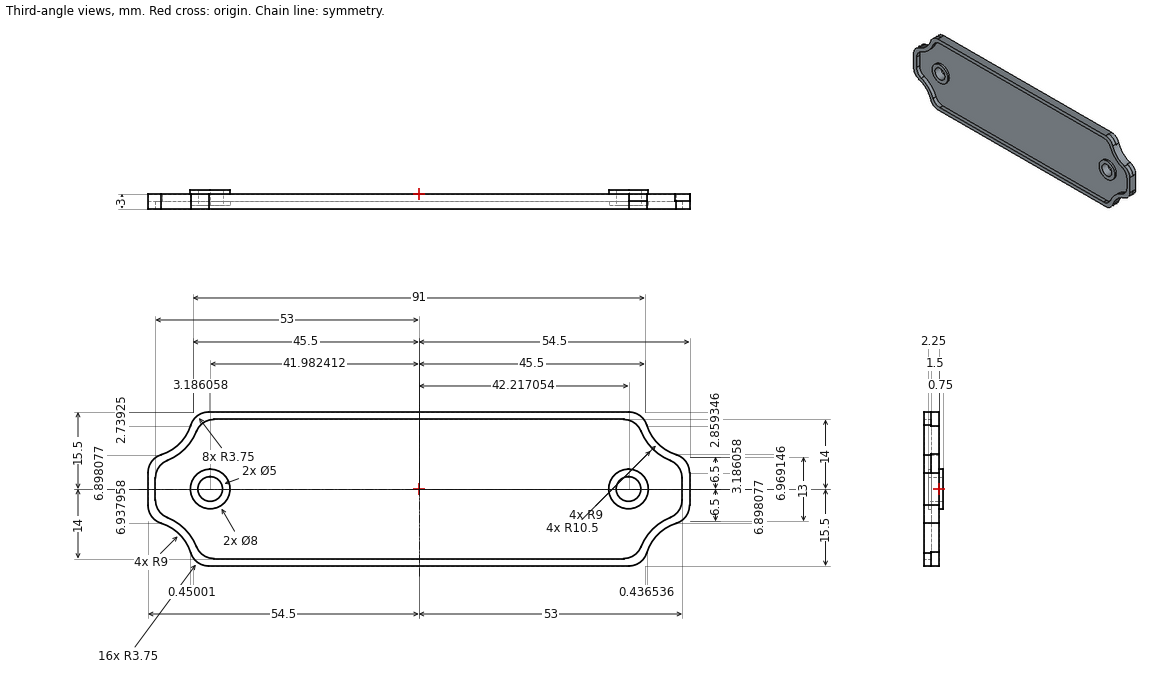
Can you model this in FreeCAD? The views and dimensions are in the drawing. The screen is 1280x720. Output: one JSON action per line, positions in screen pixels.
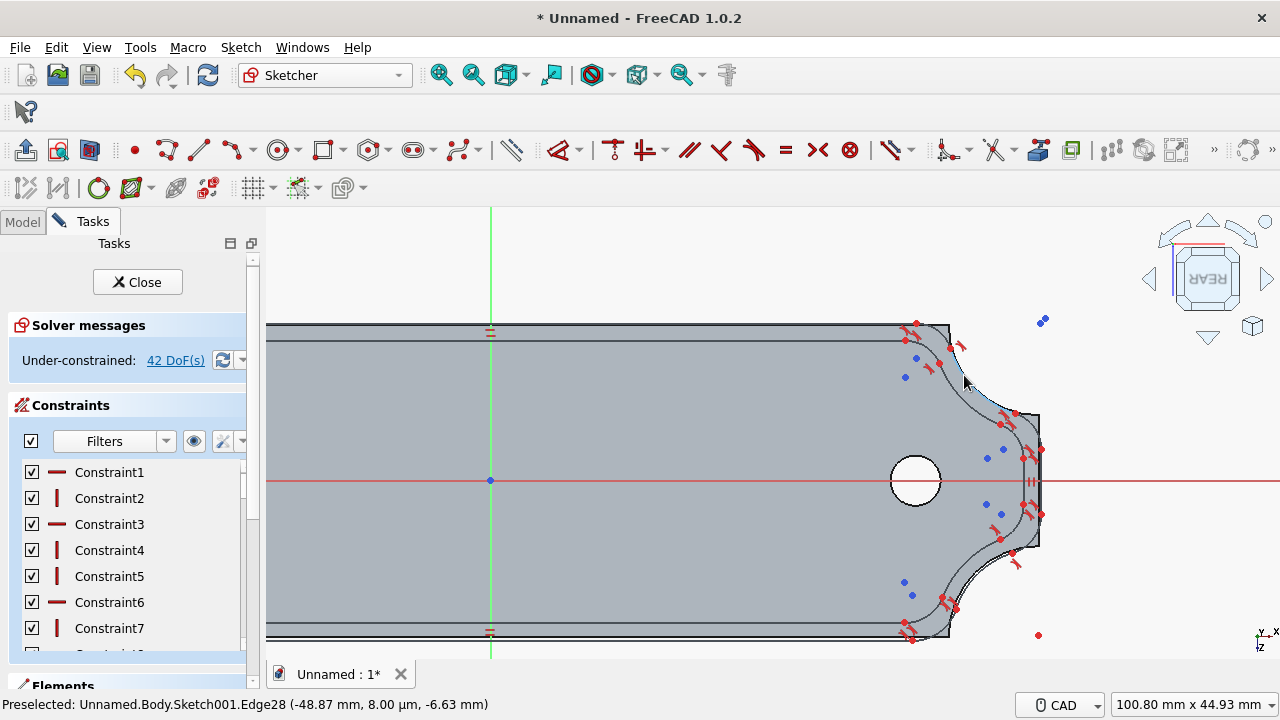
{"action": "left_click", "coordinate": [963, 374]}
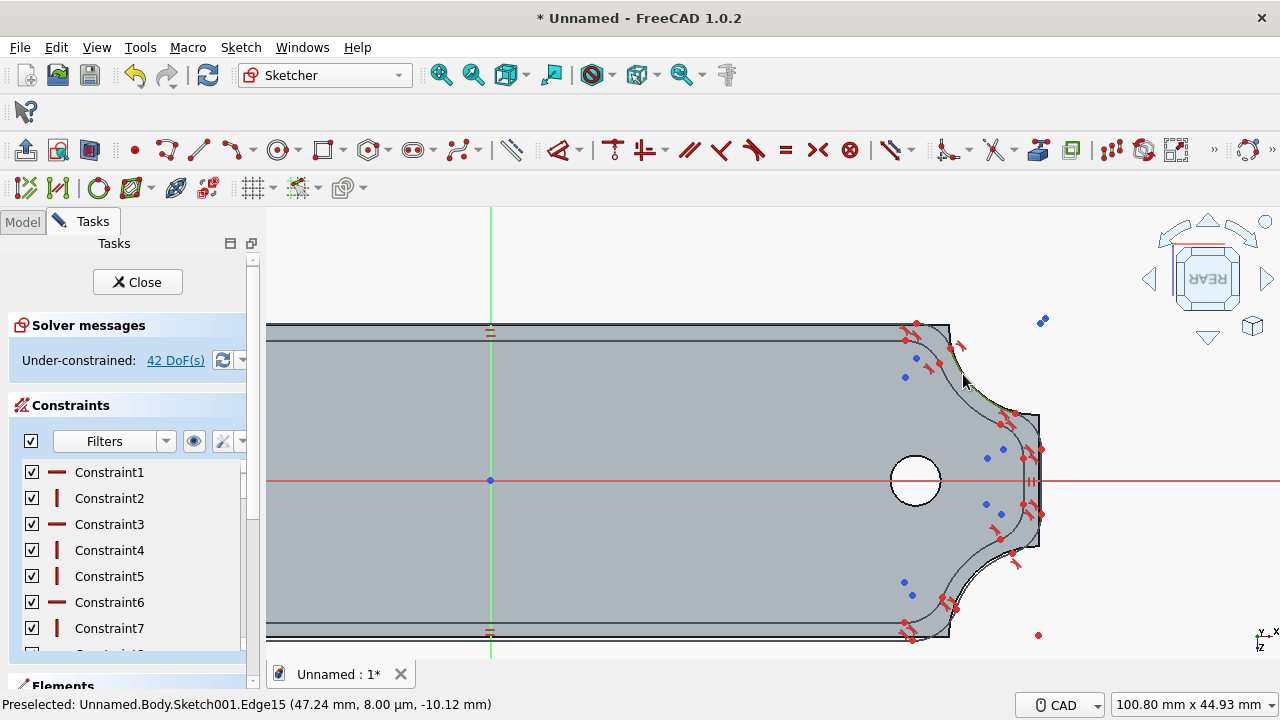
{"action": "left_click", "coordinate": [952, 387]}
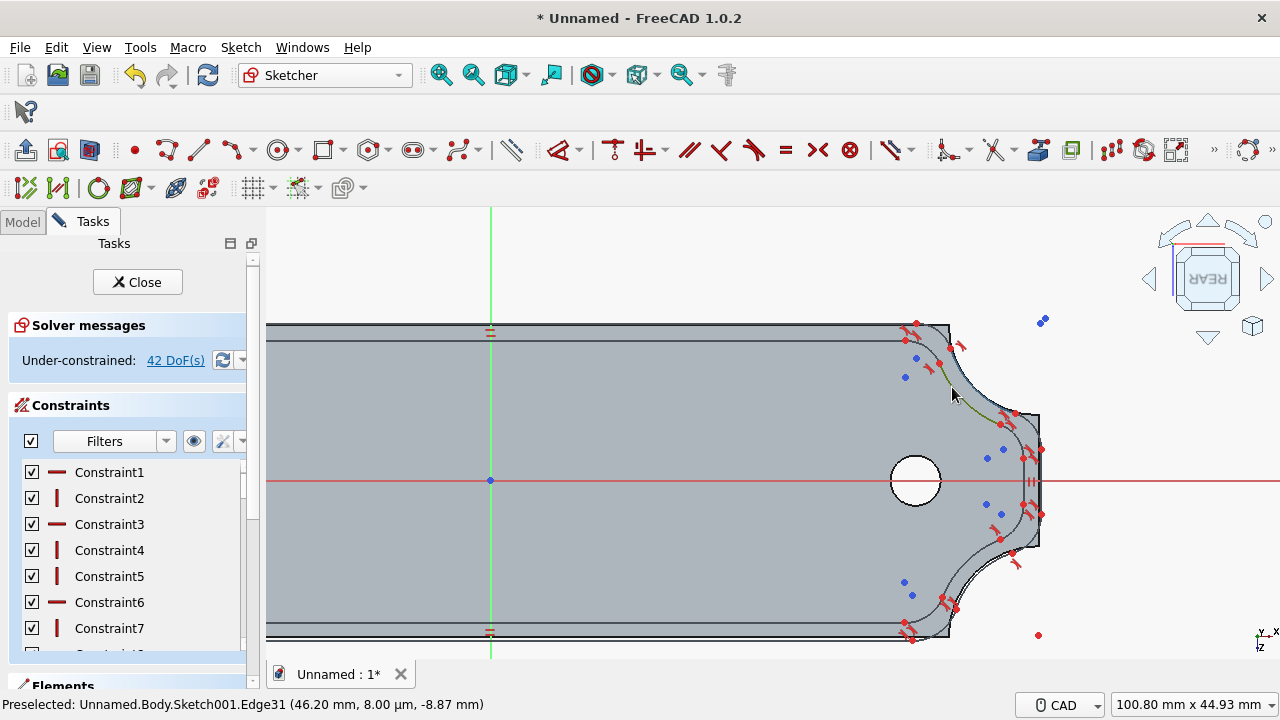
{"action": "left_click", "coordinate": [614, 150]}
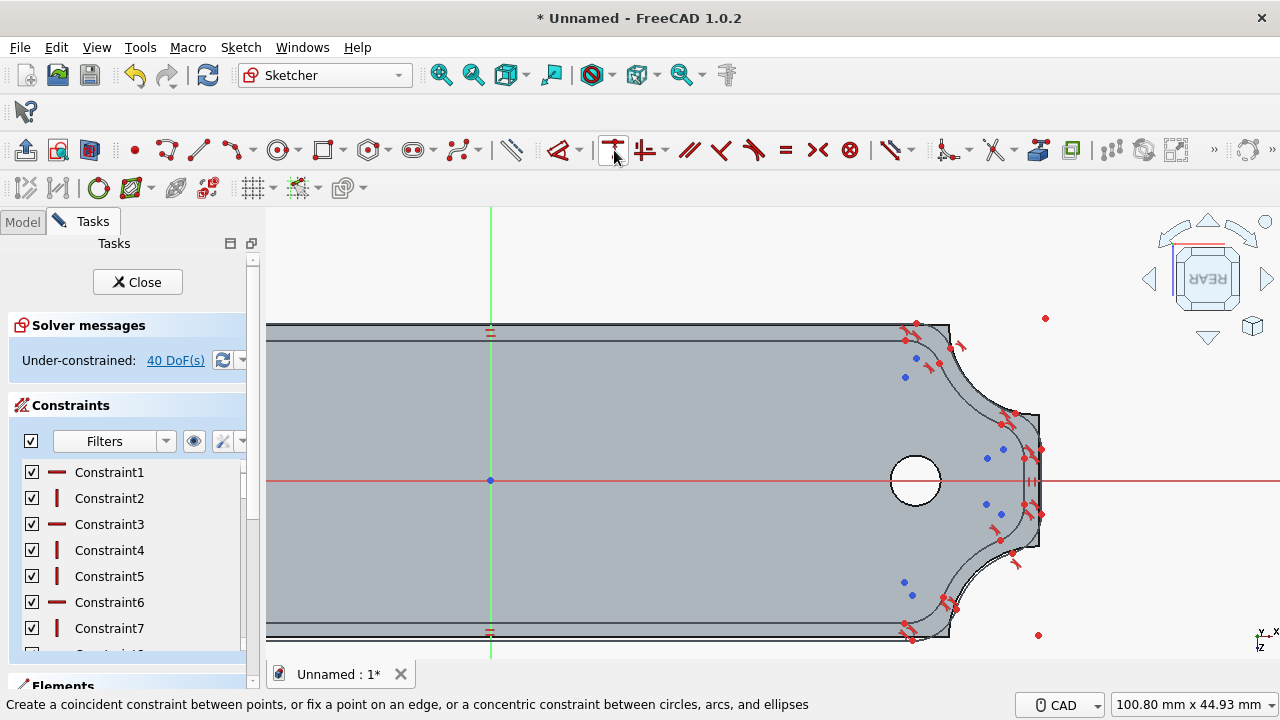
{"action": "scroll", "coordinate": [964, 375], "scroll_direction": "down", "scroll_amount": 3}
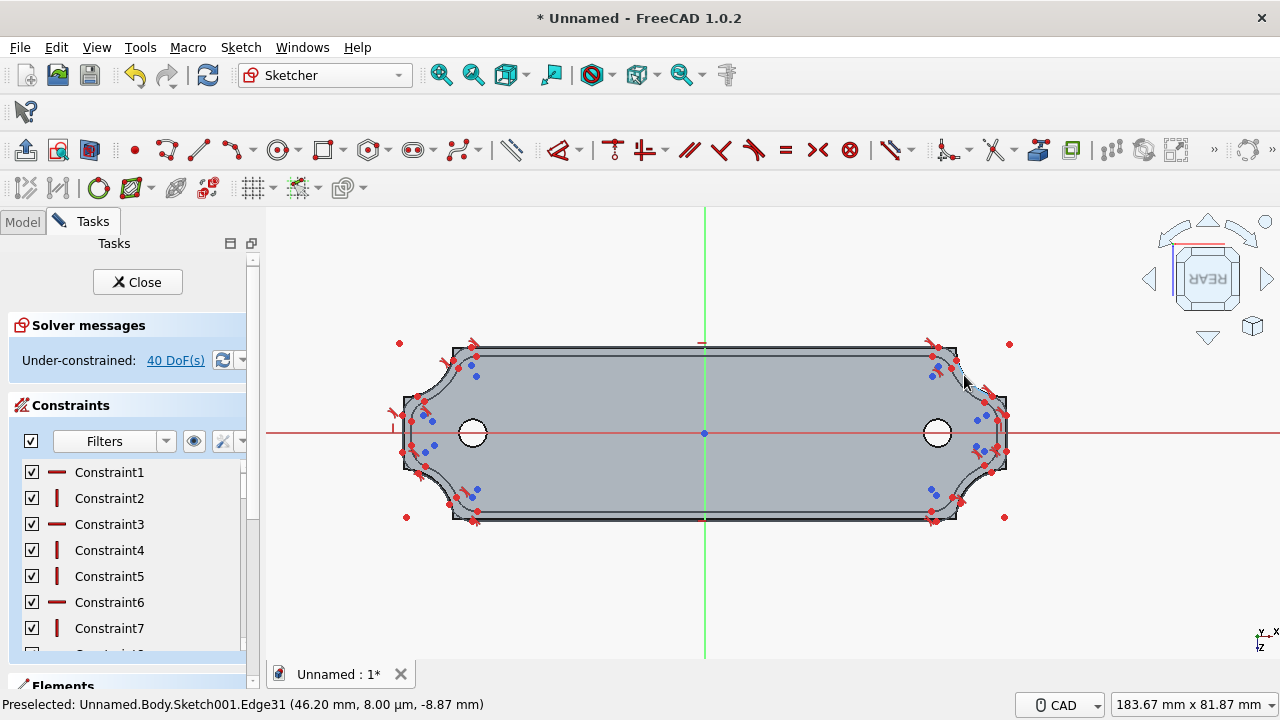
{"action": "scroll", "coordinate": [464, 348], "scroll_direction": "up", "scroll_amount": 4}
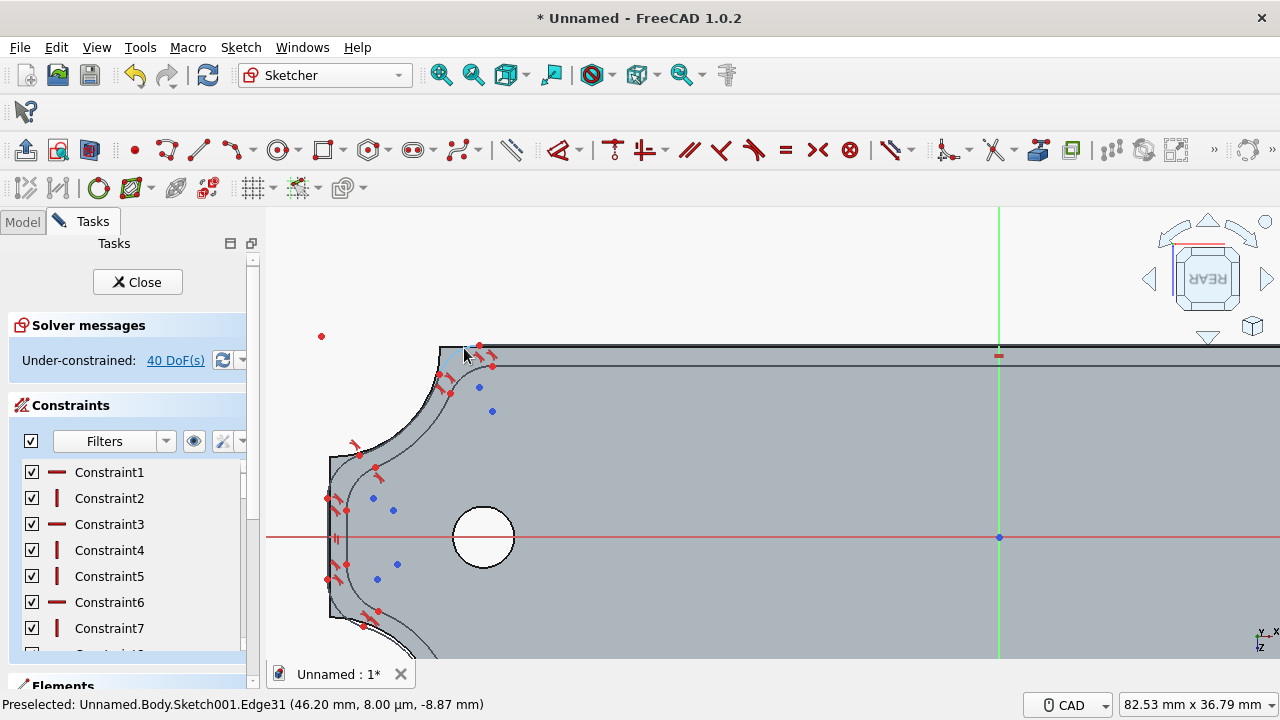
{"action": "left_click", "coordinate": [464, 348]}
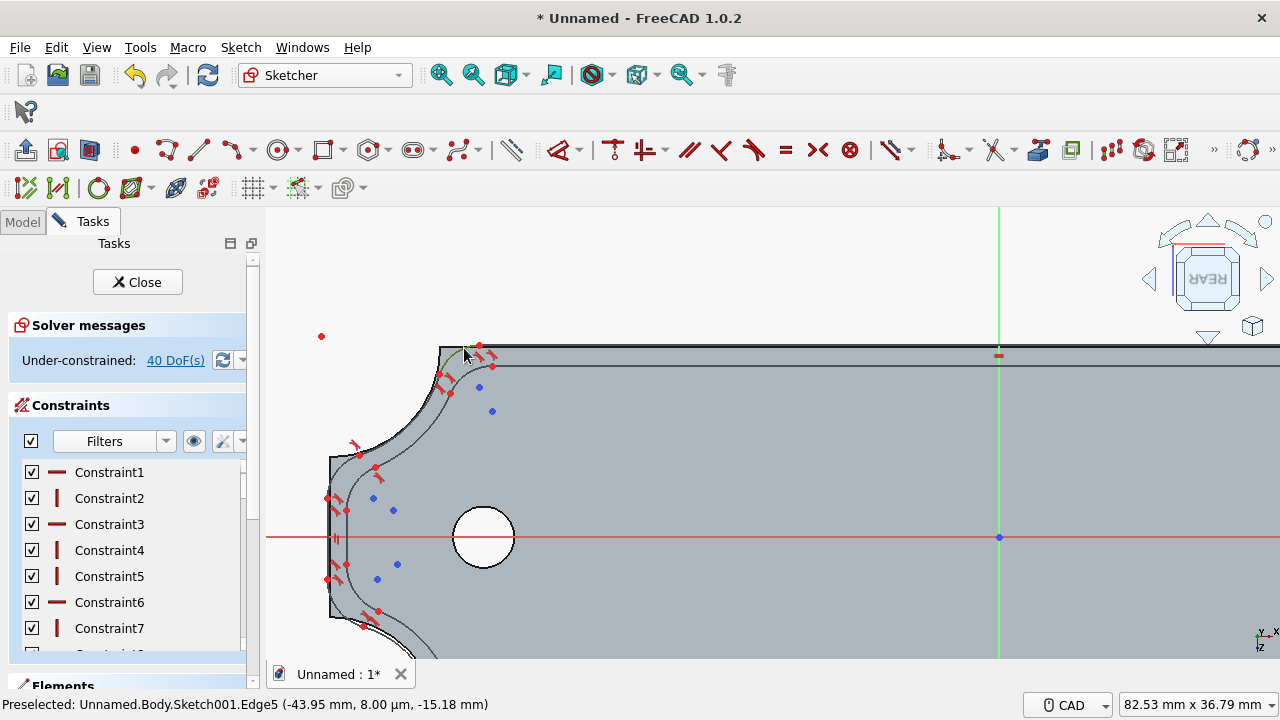
{"action": "left_click", "coordinate": [344, 463]}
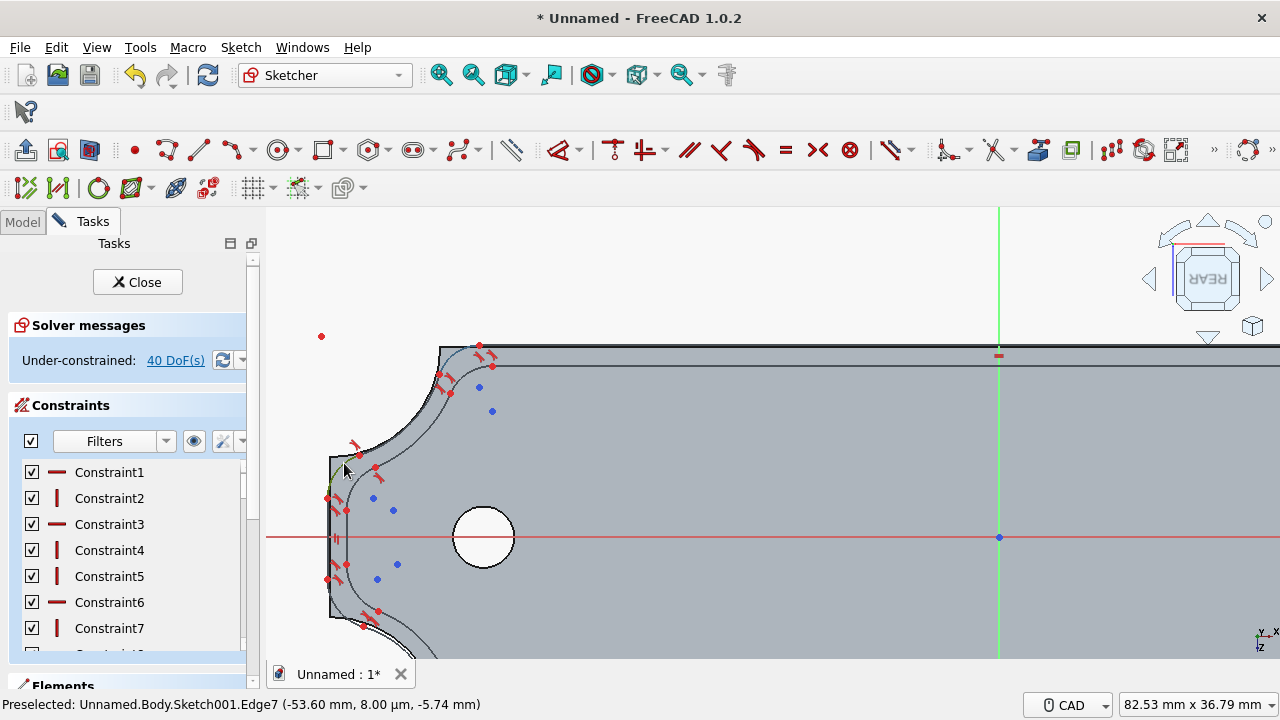
{"action": "left_click", "coordinate": [331, 598]}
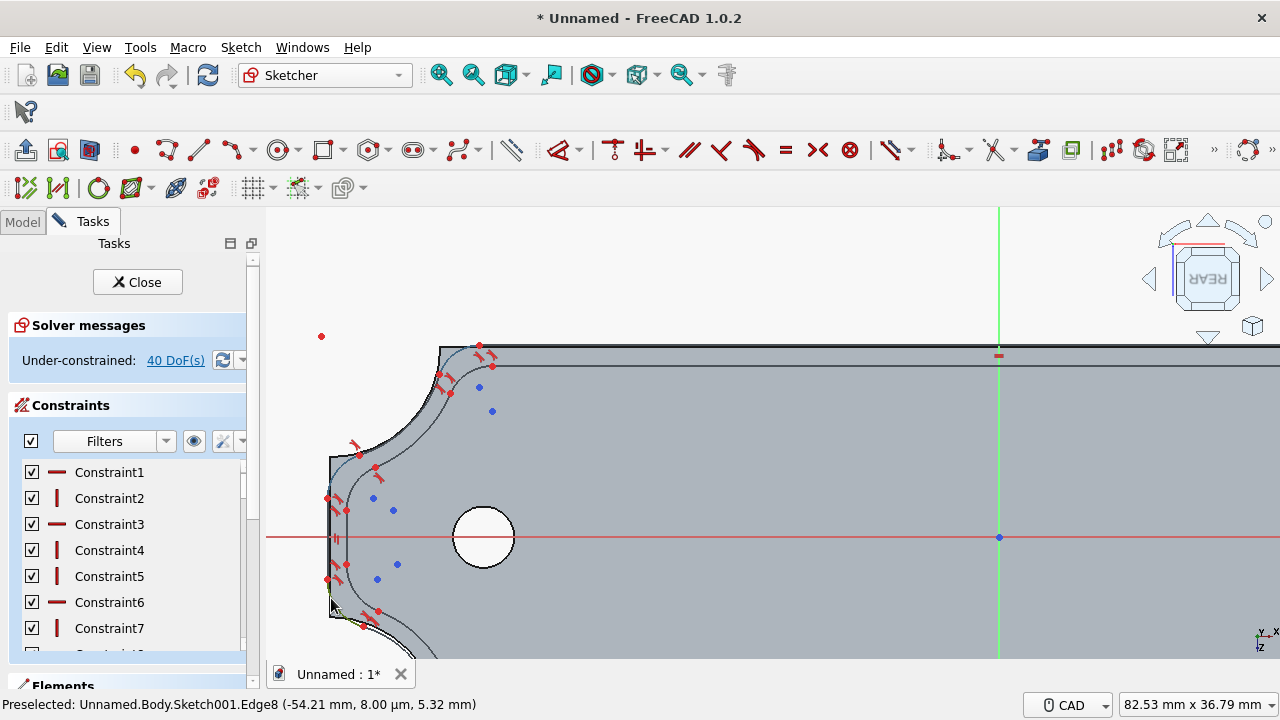
{"action": "scroll", "coordinate": [464, 348], "scroll_direction": "down", "scroll_amount": 4}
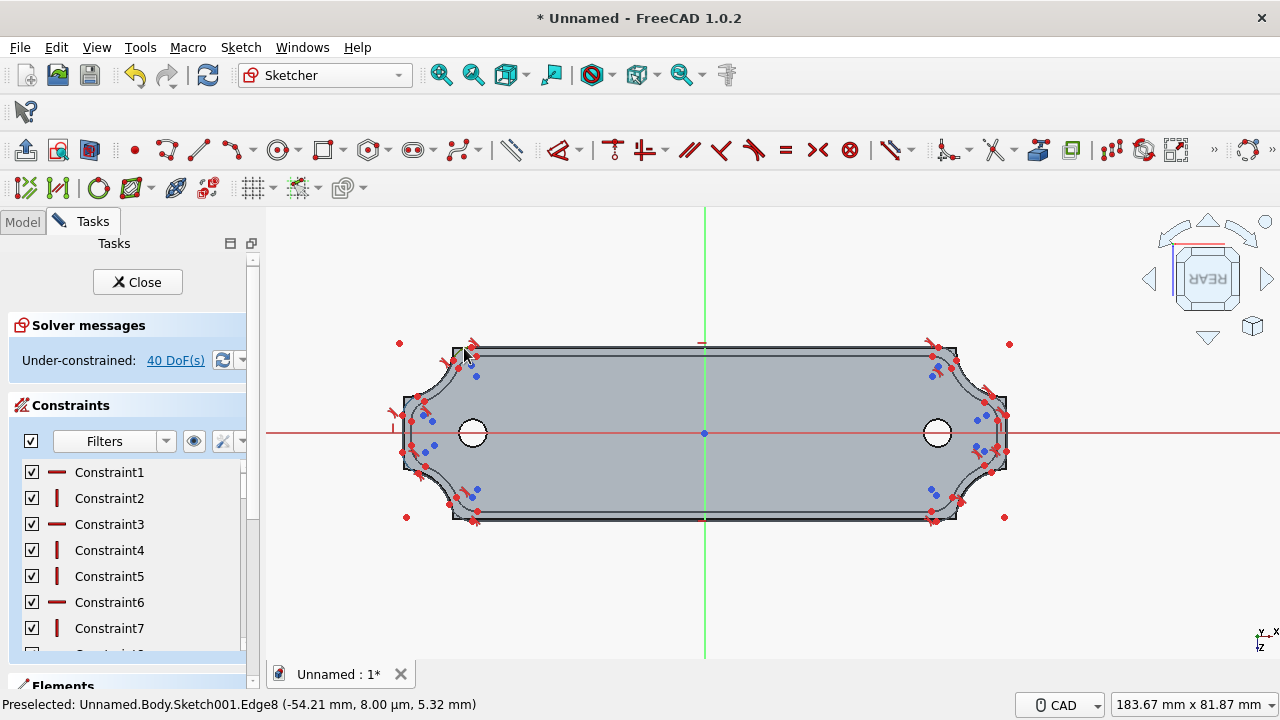
{"action": "scroll", "coordinate": [454, 512], "scroll_direction": "up", "scroll_amount": 3}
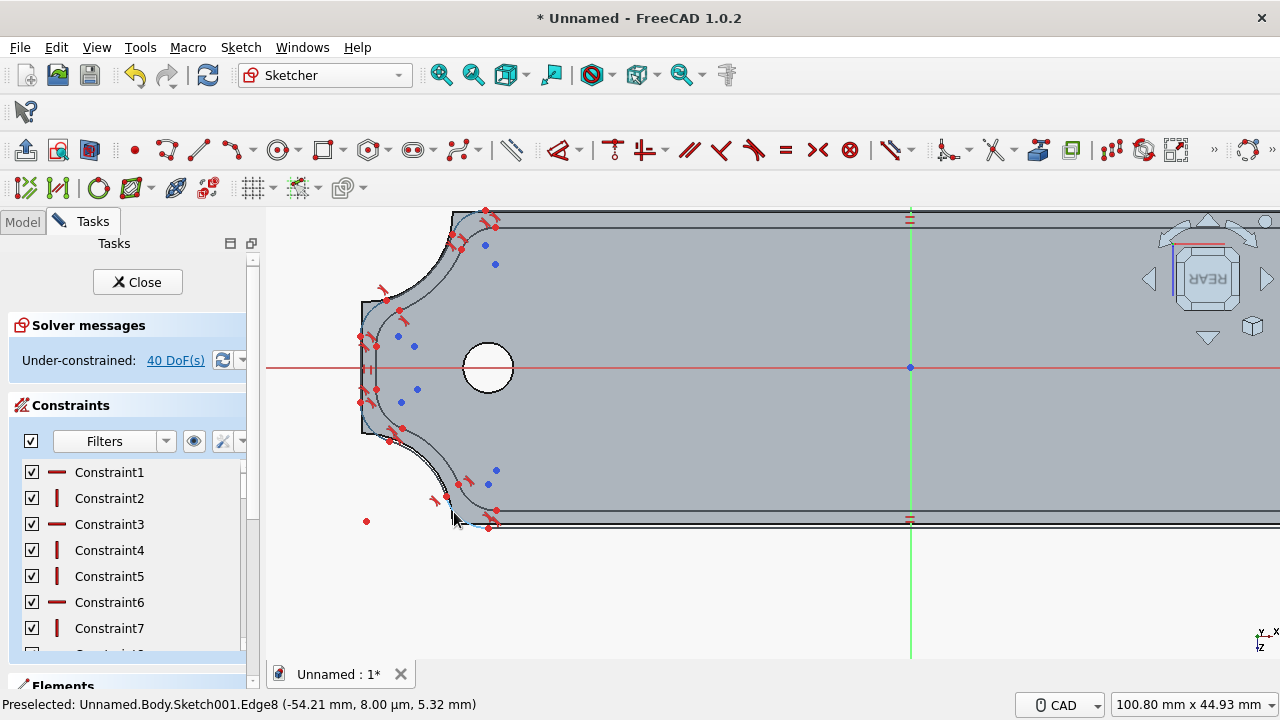
{"action": "left_click", "coordinate": [454, 512]}